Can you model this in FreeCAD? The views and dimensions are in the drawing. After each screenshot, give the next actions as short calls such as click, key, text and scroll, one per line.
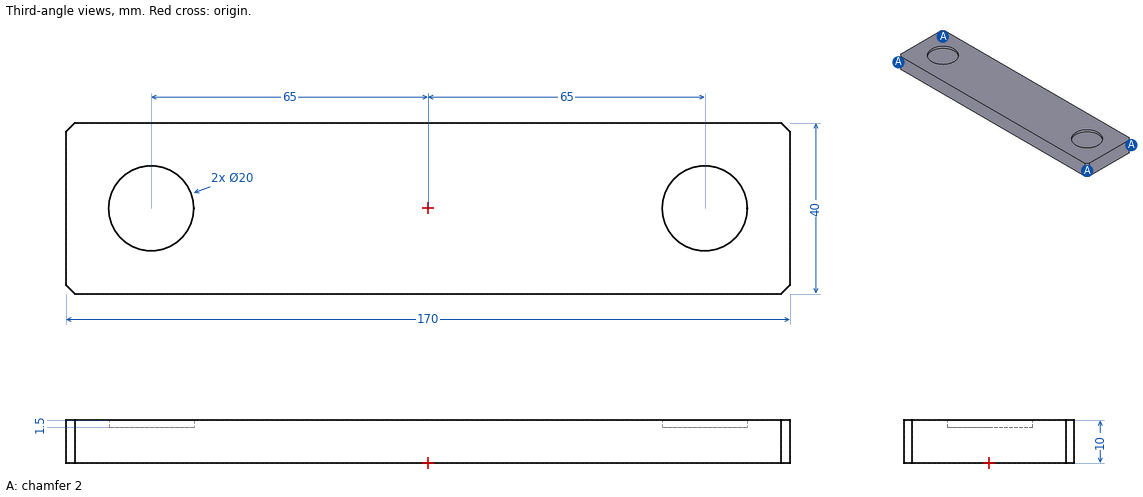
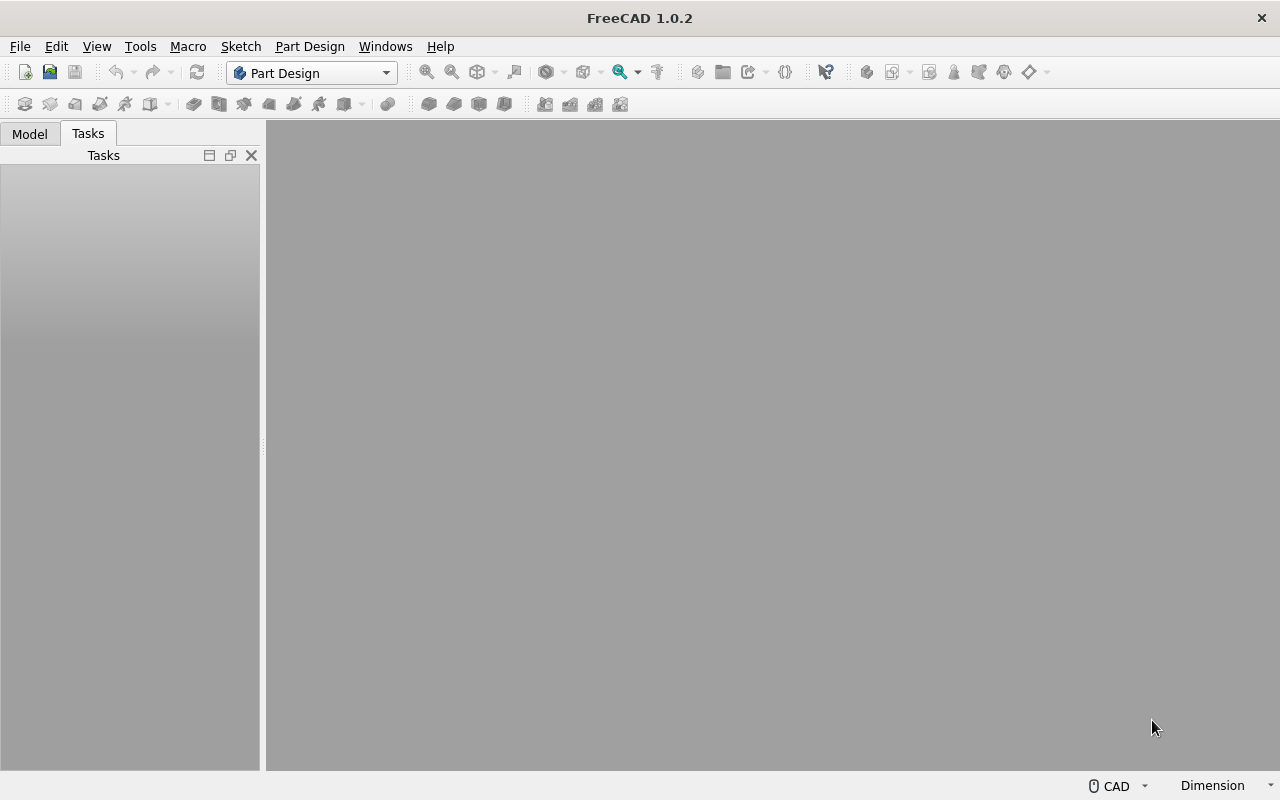
key(ctrl+n)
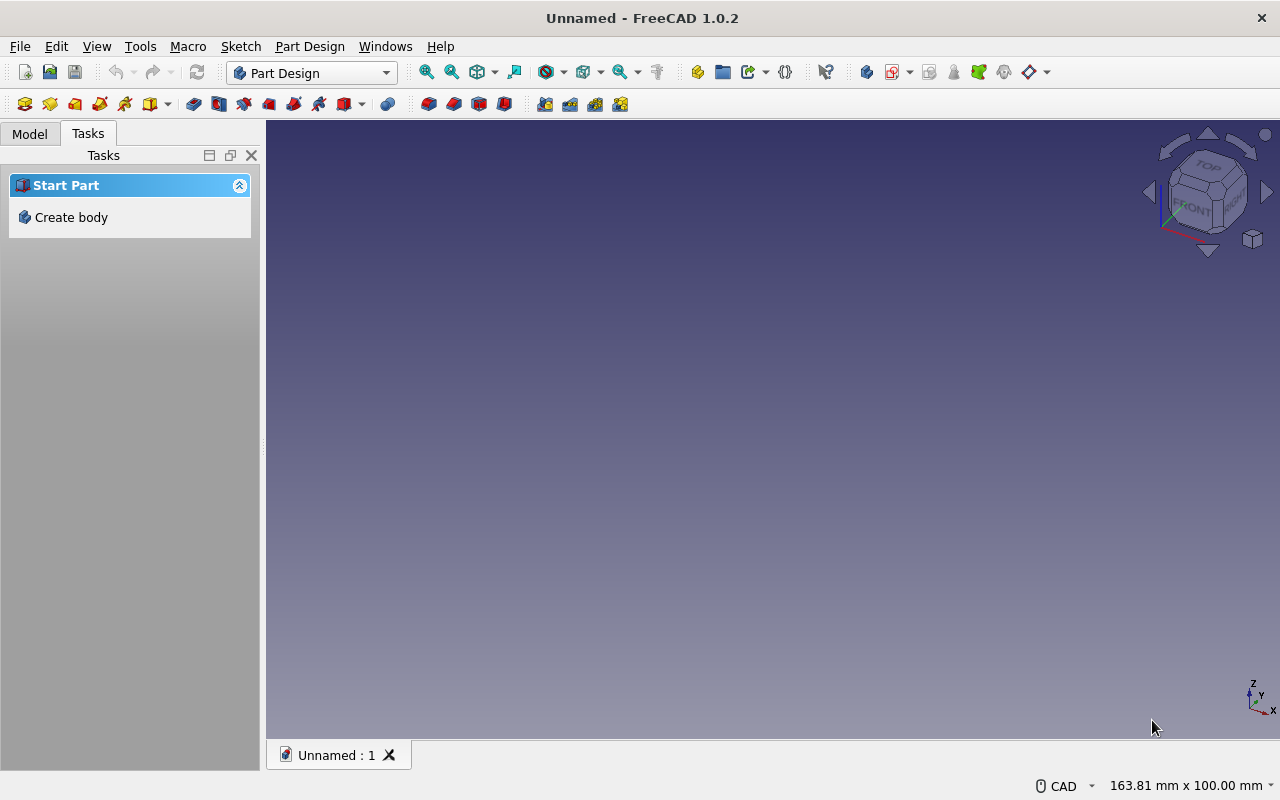
click(892, 72)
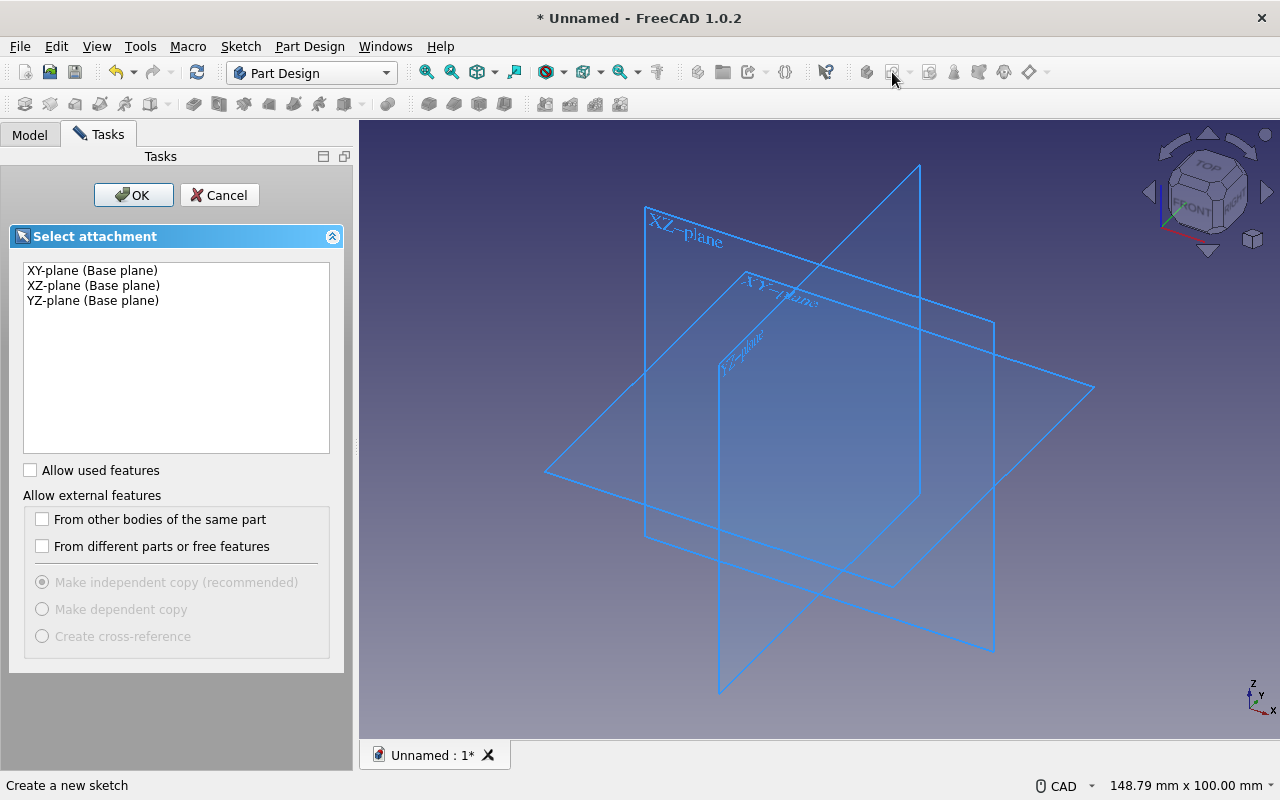
click(84, 270)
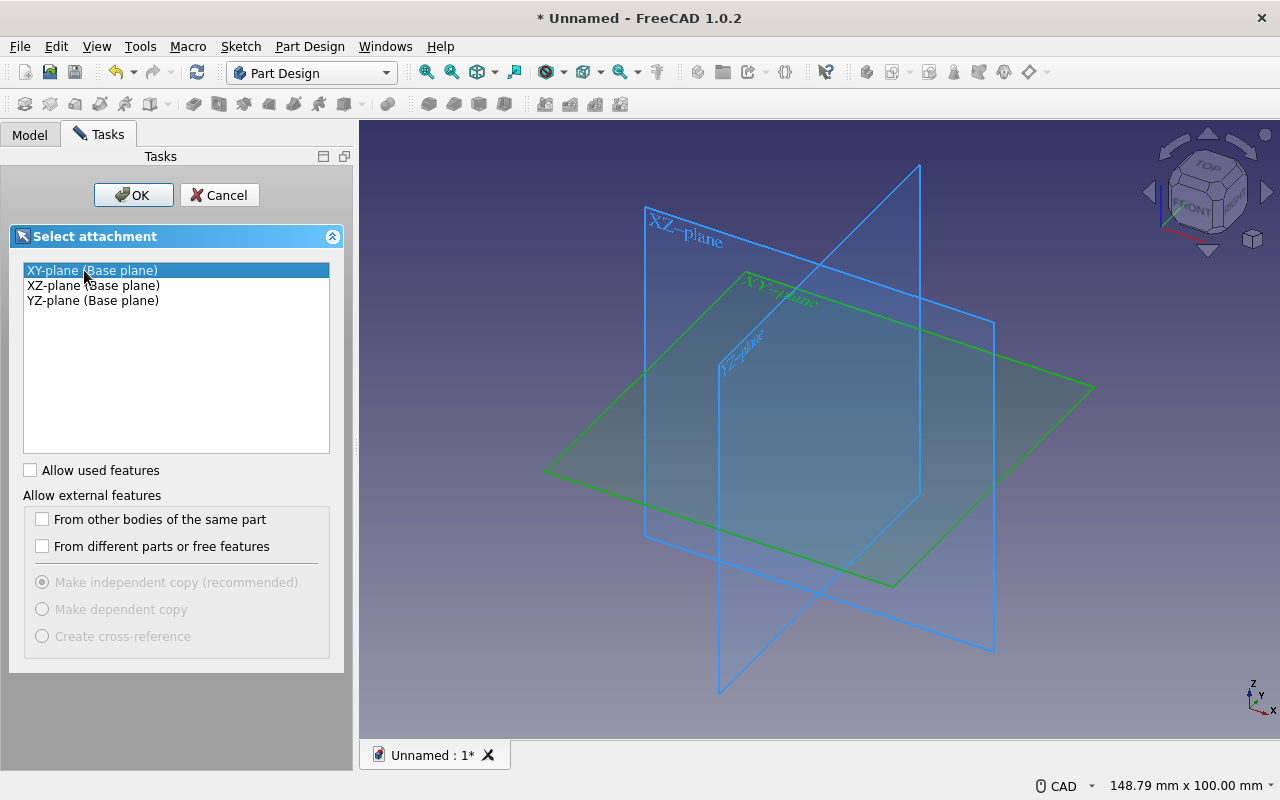
click(134, 195)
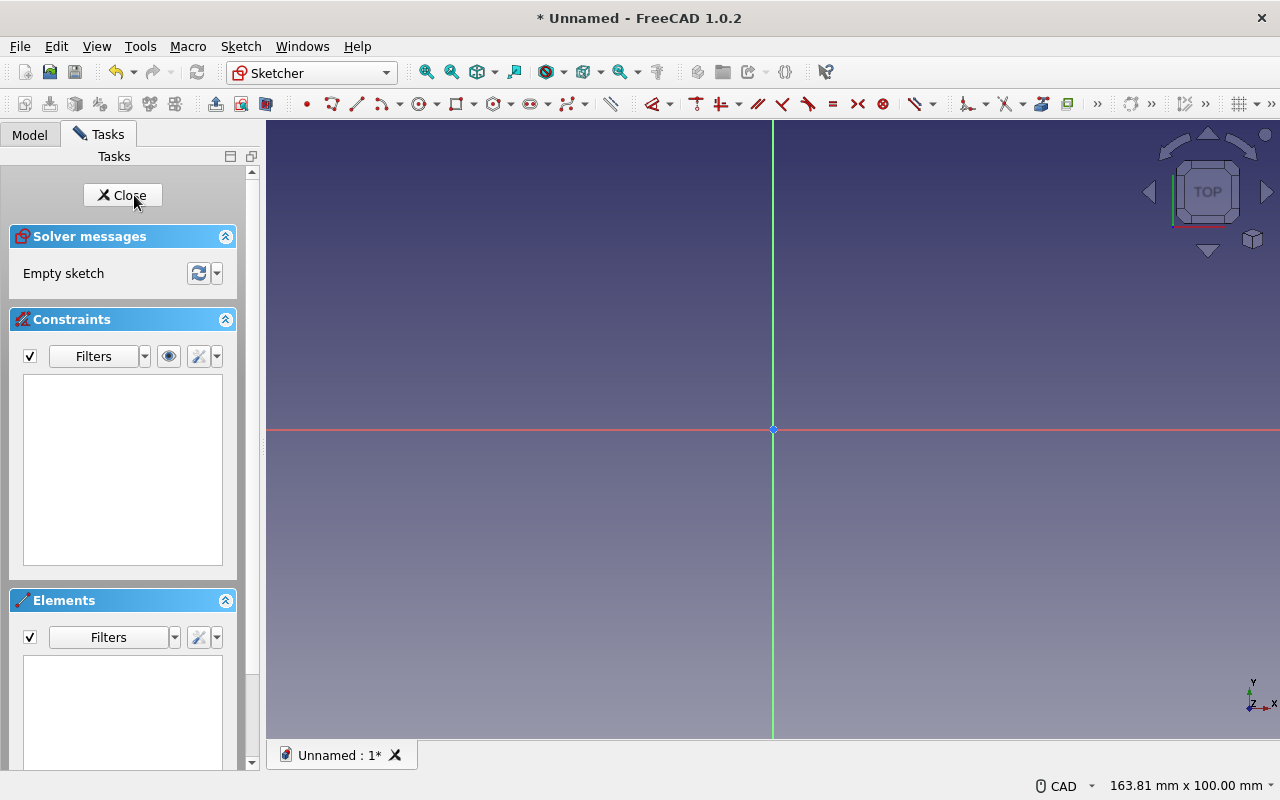
scroll(621, 430, down, 3)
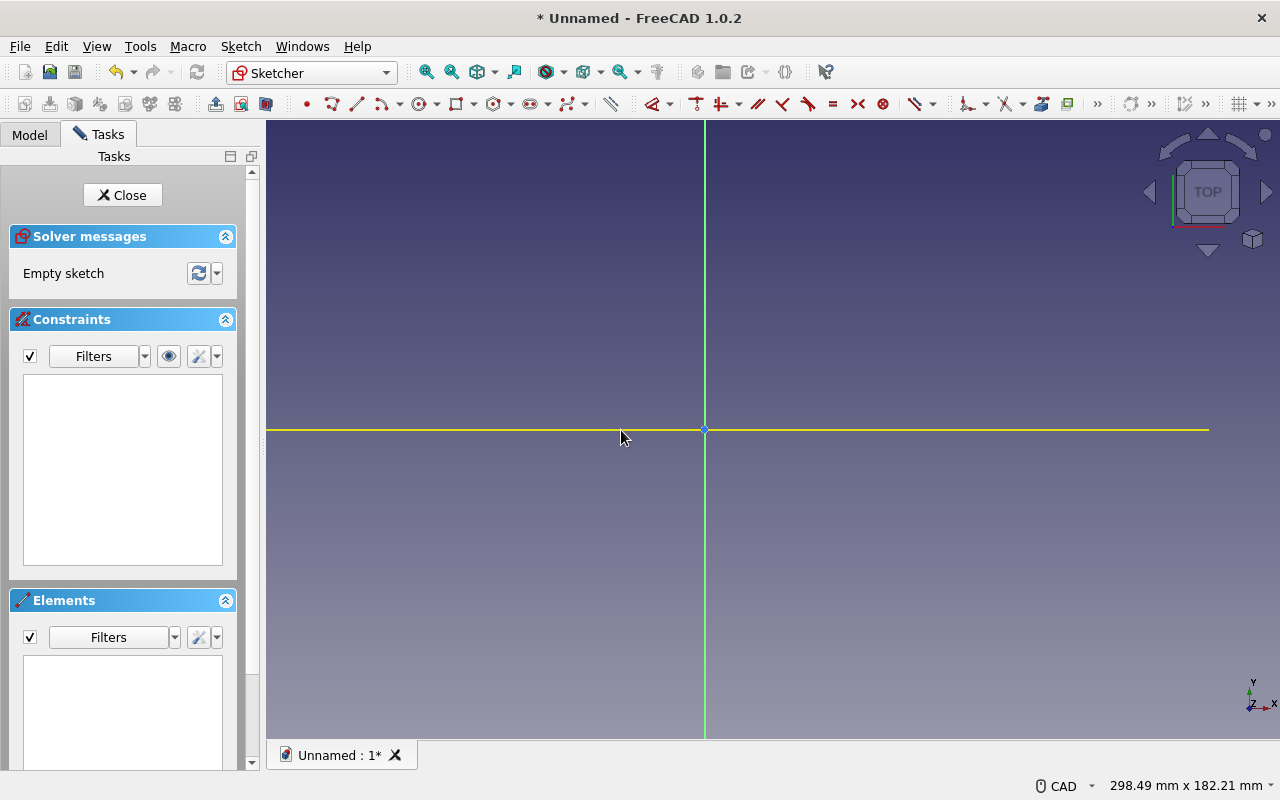
key(g)
key(v)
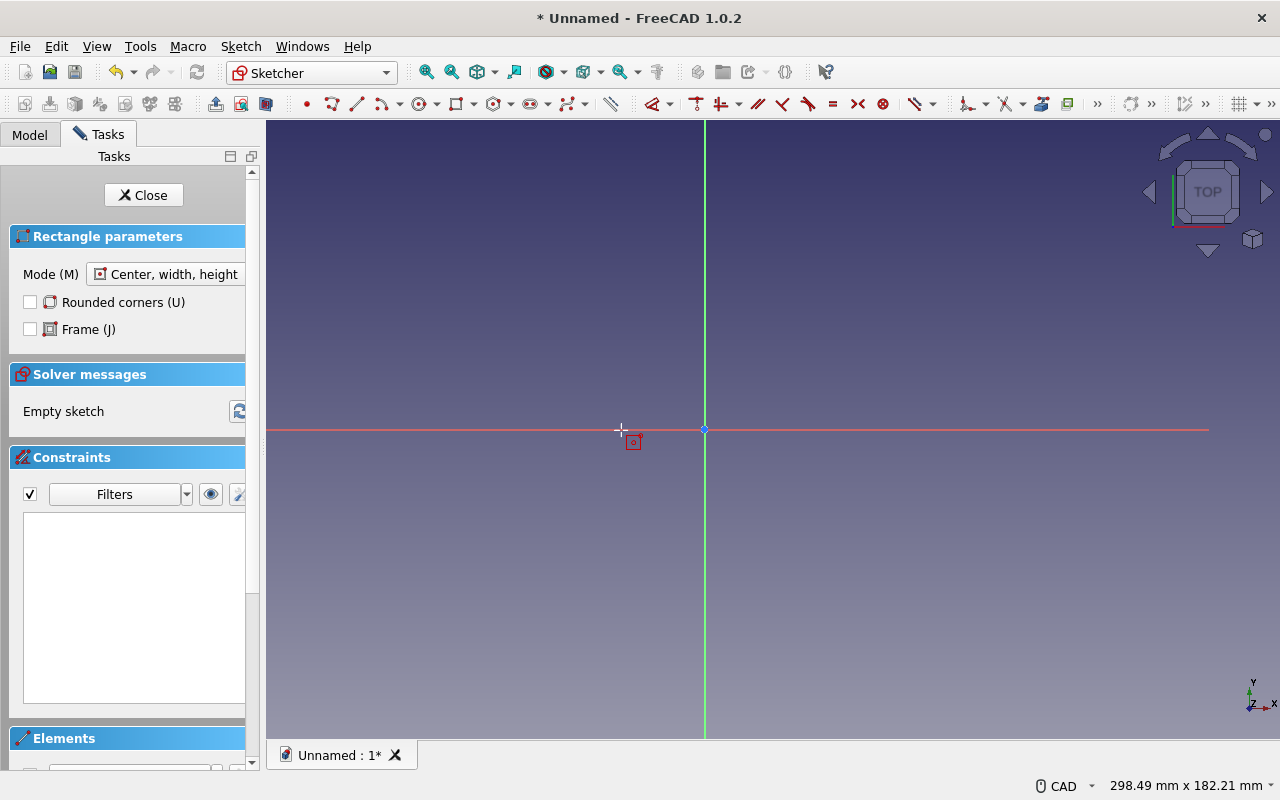
click(705, 430)
click(993, 362)
key(Escape)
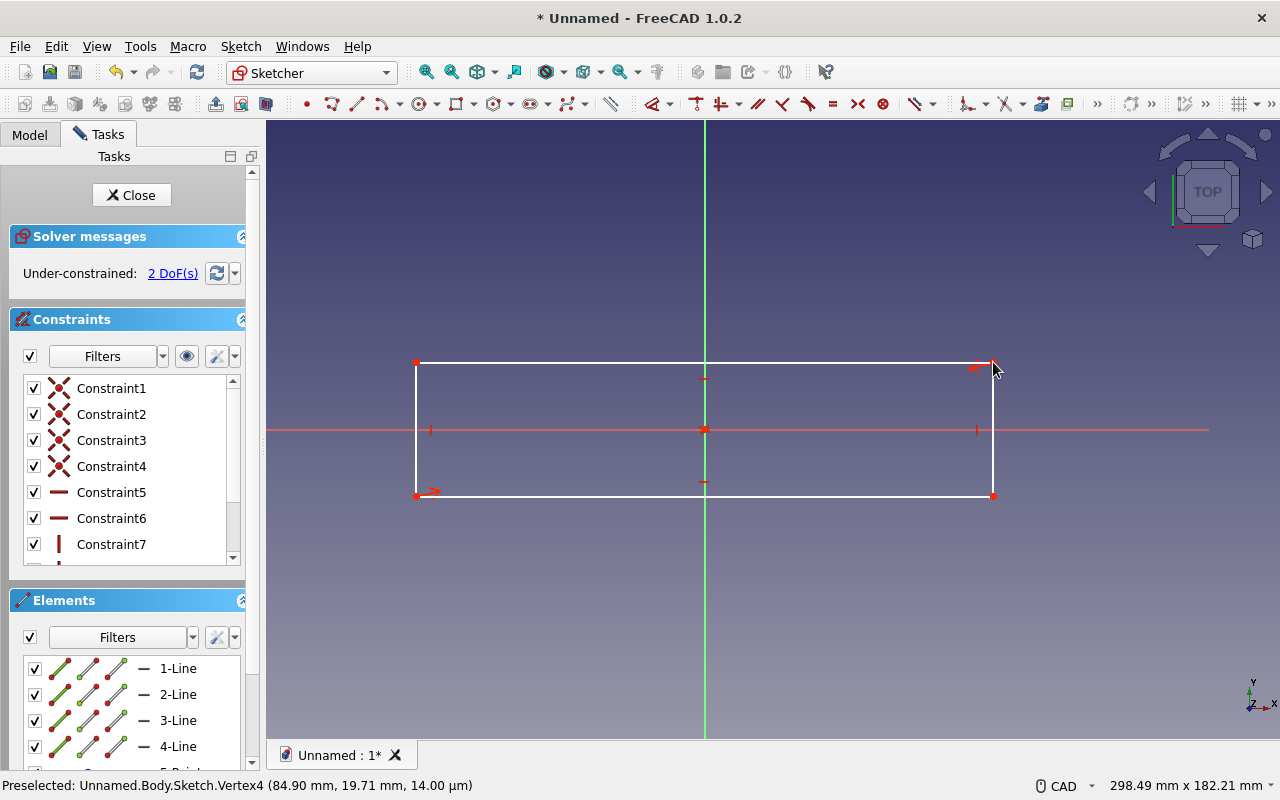
key(d)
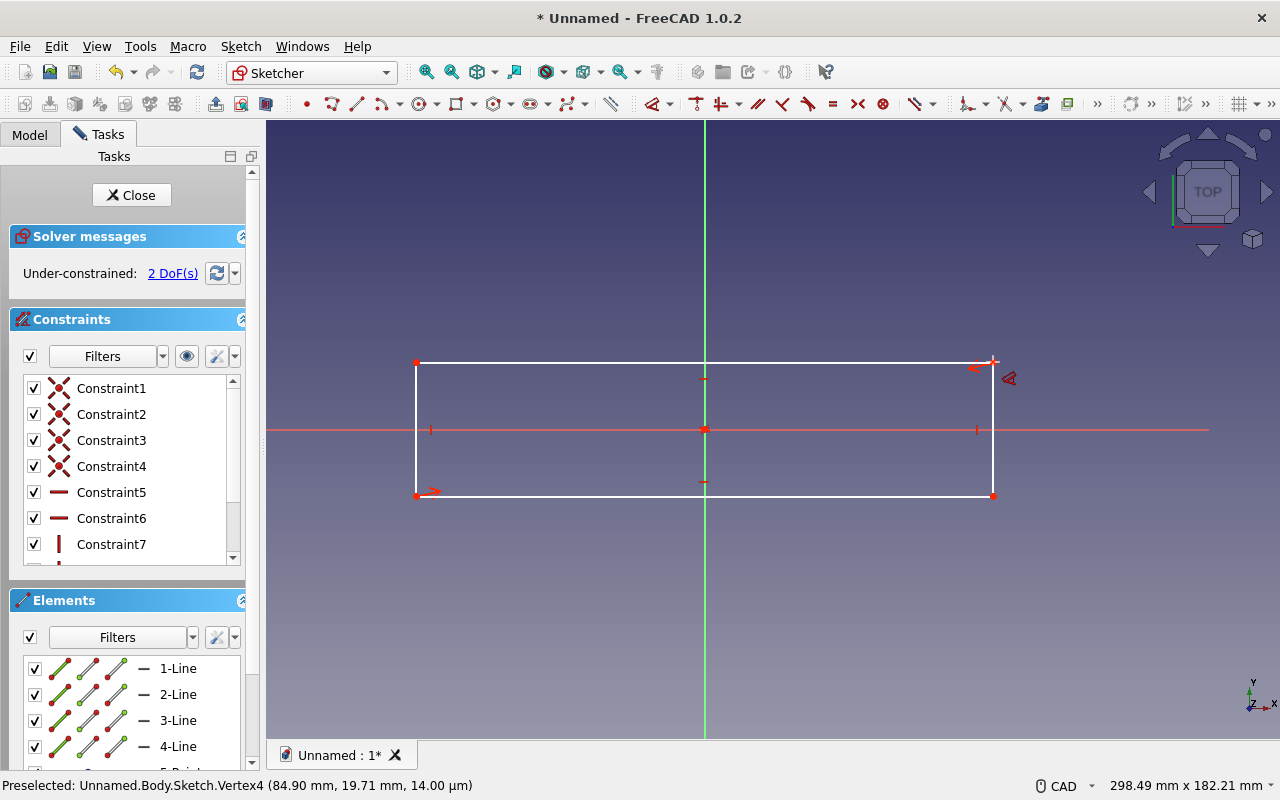
click(993, 457)
click(1027, 399)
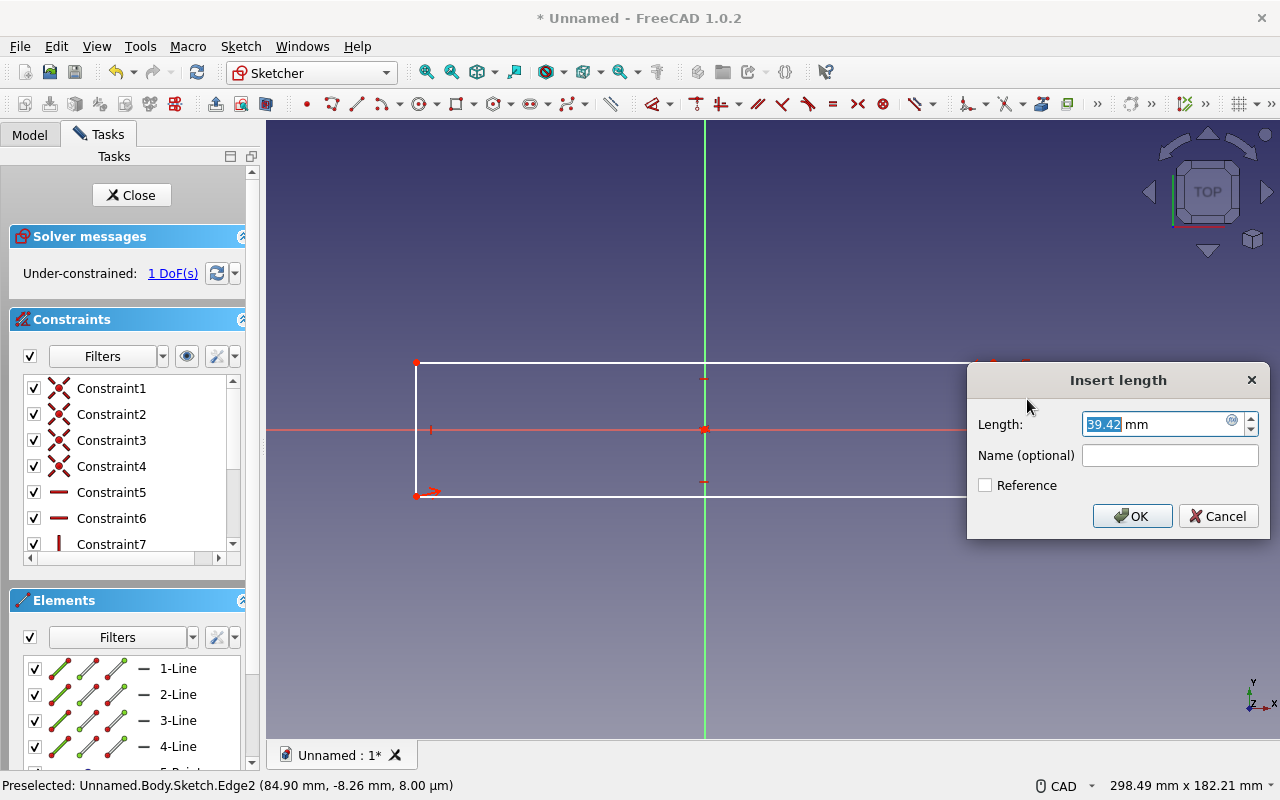
text(40)
key(Return)